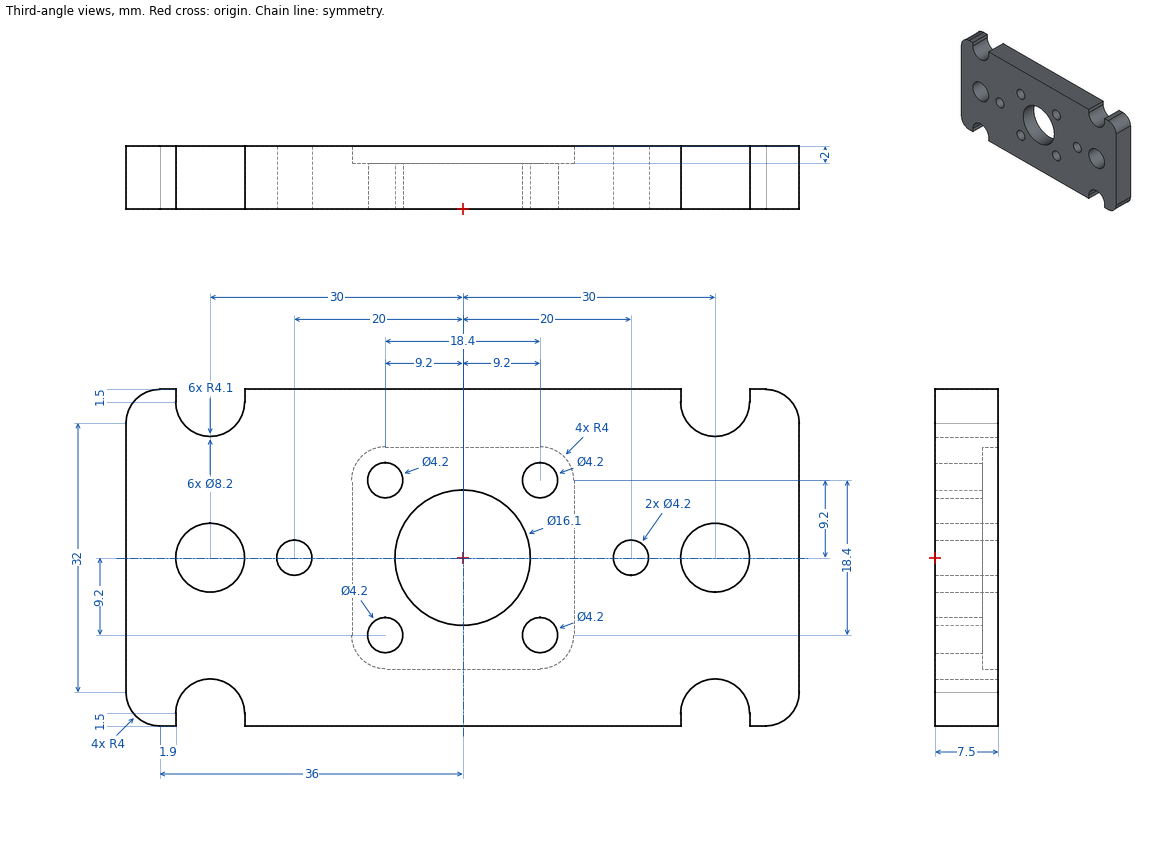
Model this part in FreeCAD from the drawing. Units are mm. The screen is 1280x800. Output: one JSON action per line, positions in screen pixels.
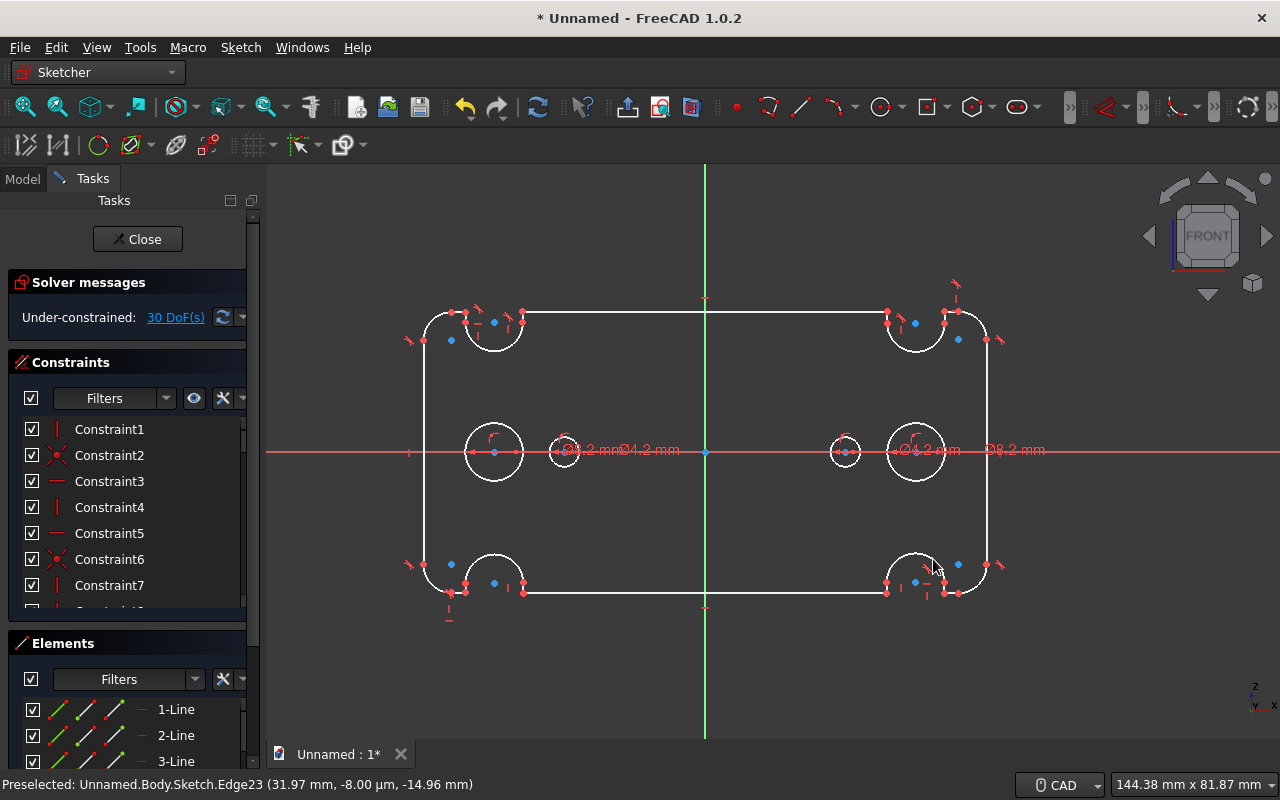
{"action": "scroll", "coordinate": [887, 588], "scroll_direction": "up", "scroll_amount": 5}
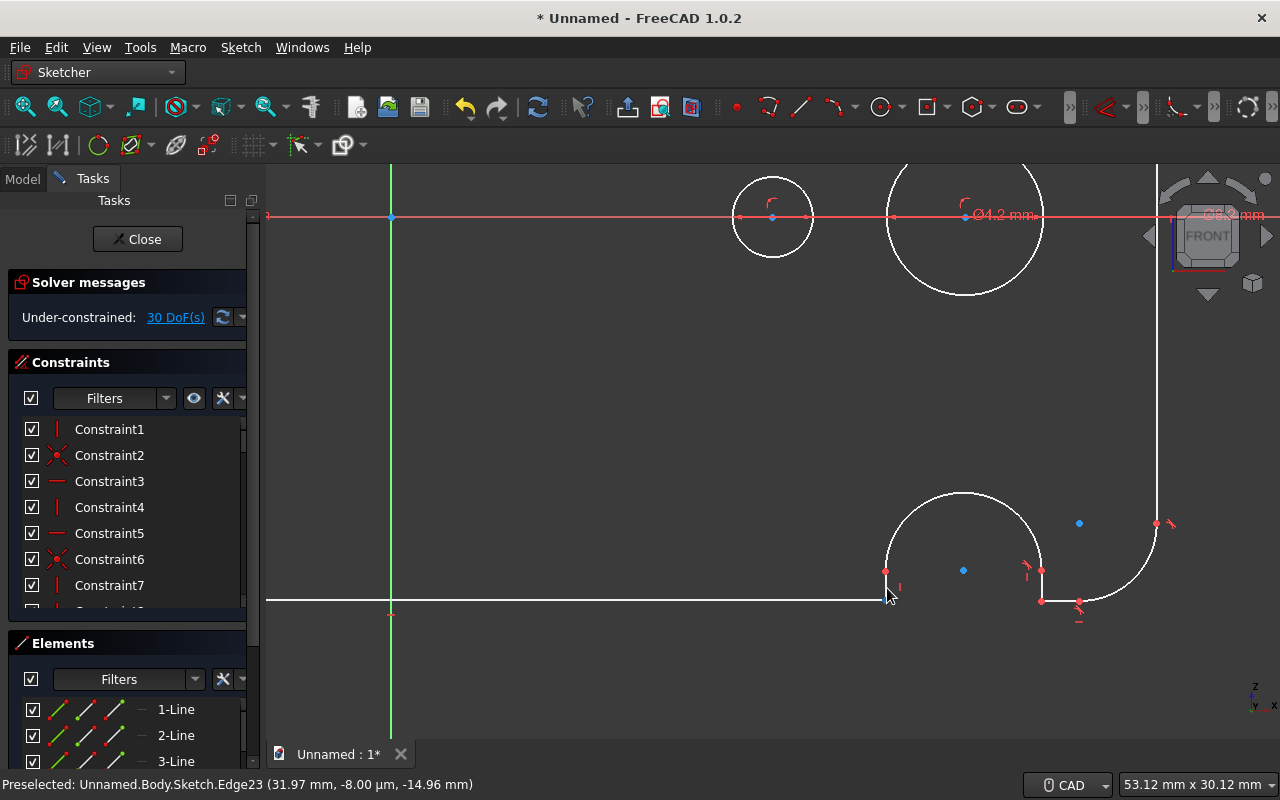
{"action": "left_click", "coordinate": [886, 586]}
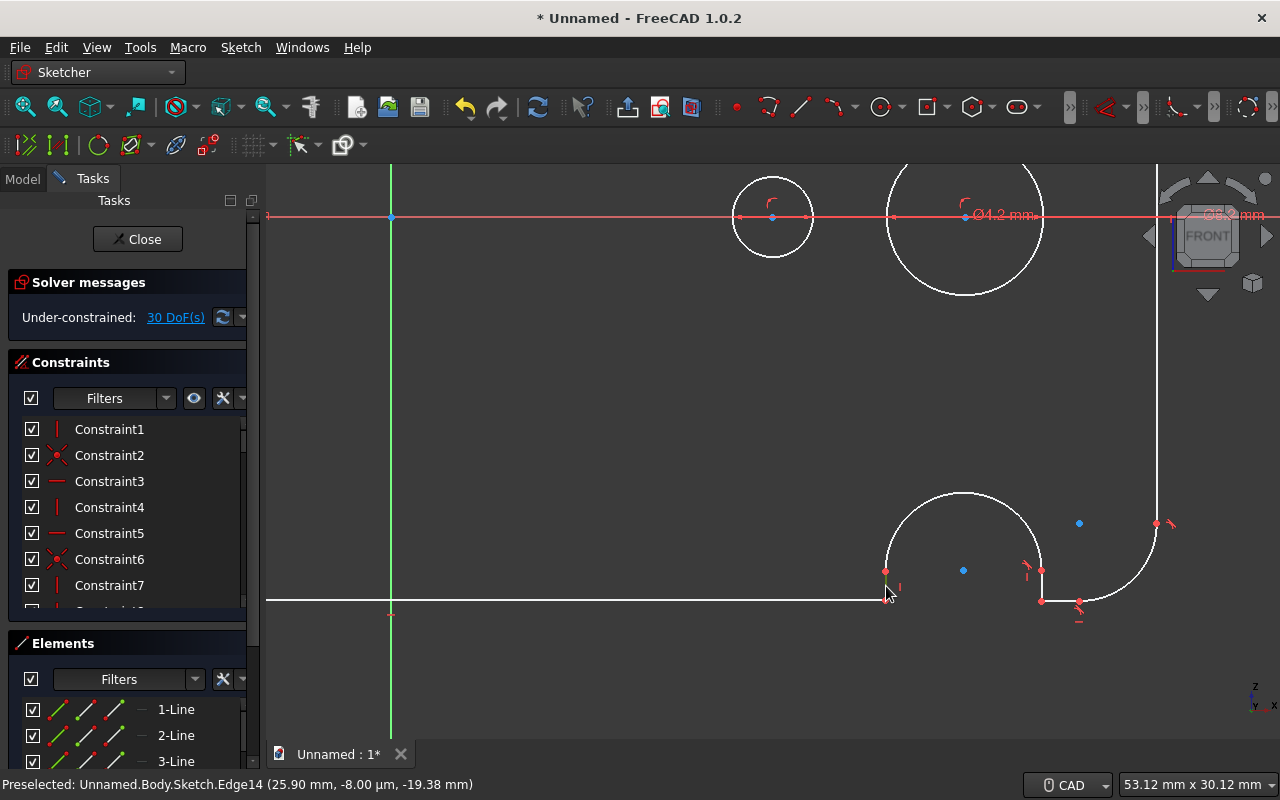
{"action": "left_click", "coordinate": [1009, 507]}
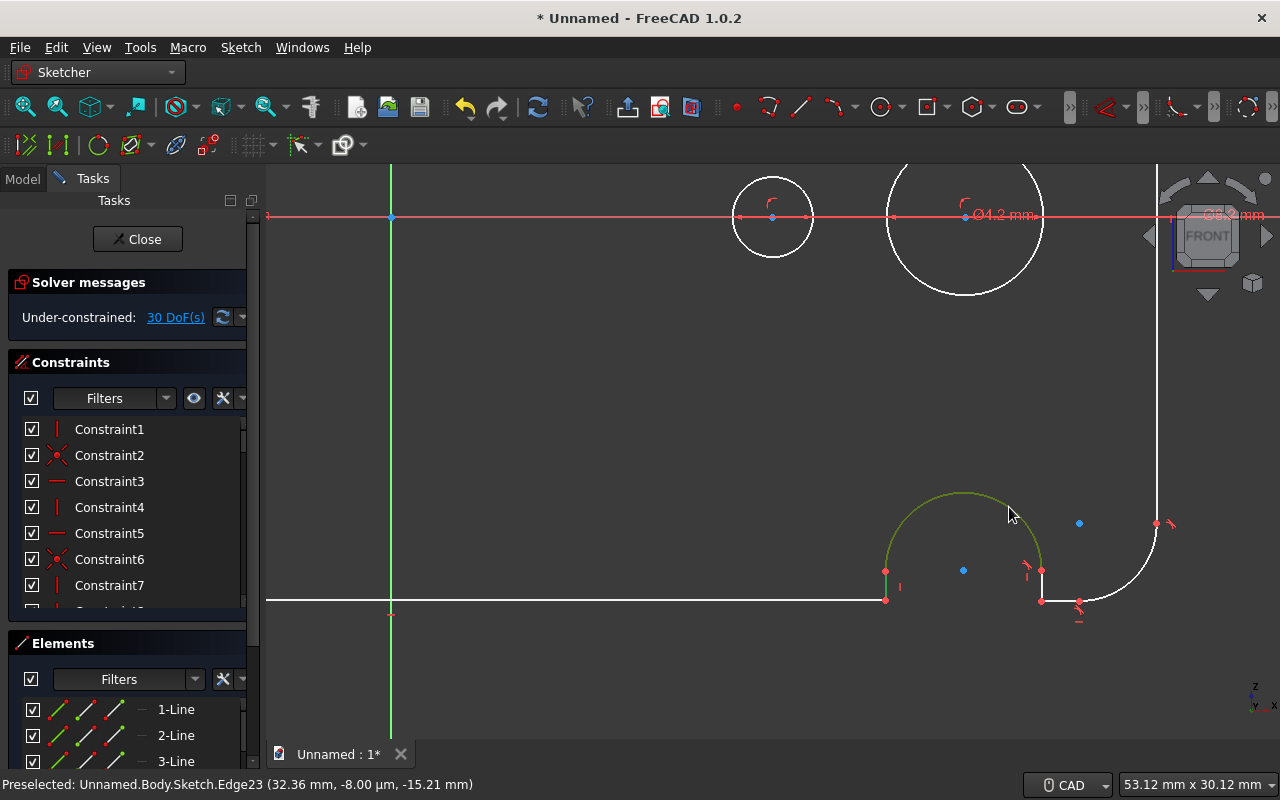
{"action": "key", "text": "t"}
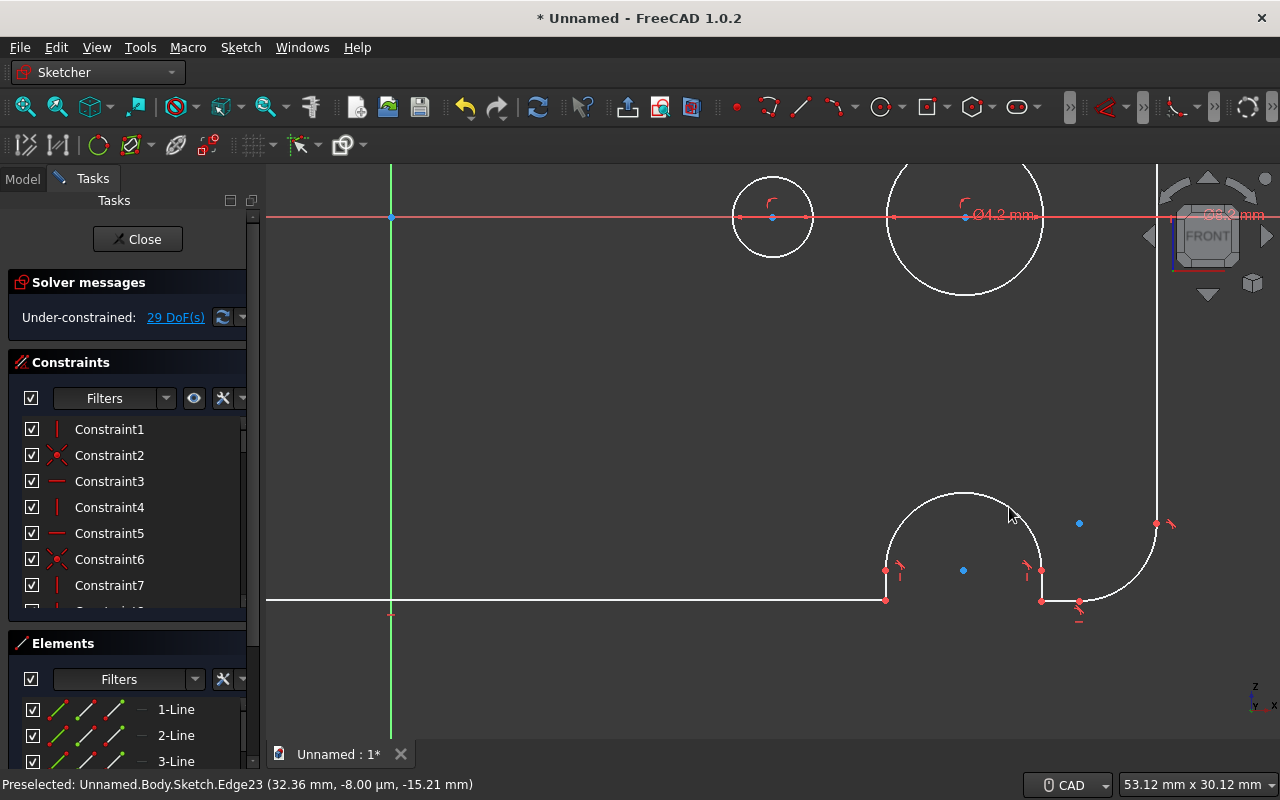
{"action": "scroll", "coordinate": [887, 588], "scroll_direction": "down", "scroll_amount": 5}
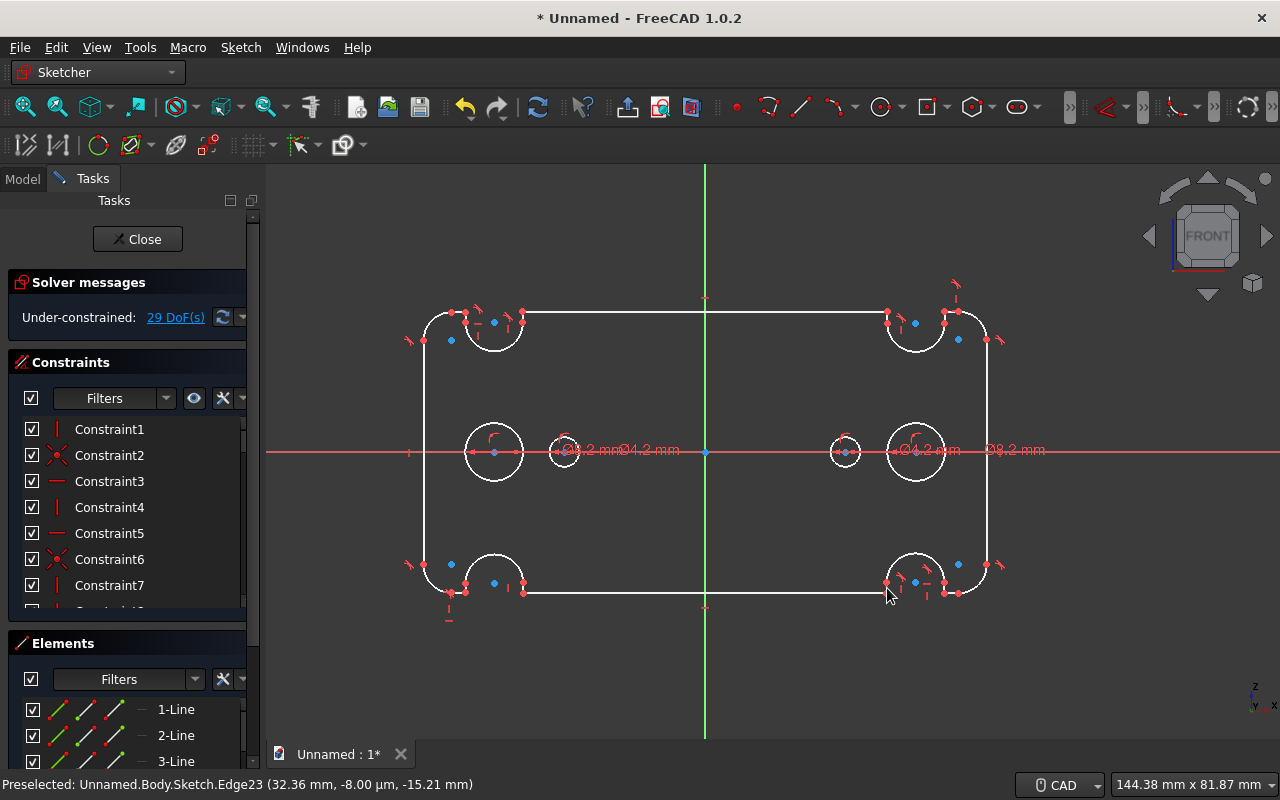
{"action": "scroll", "coordinate": [523, 589], "scroll_direction": "up", "scroll_amount": 6}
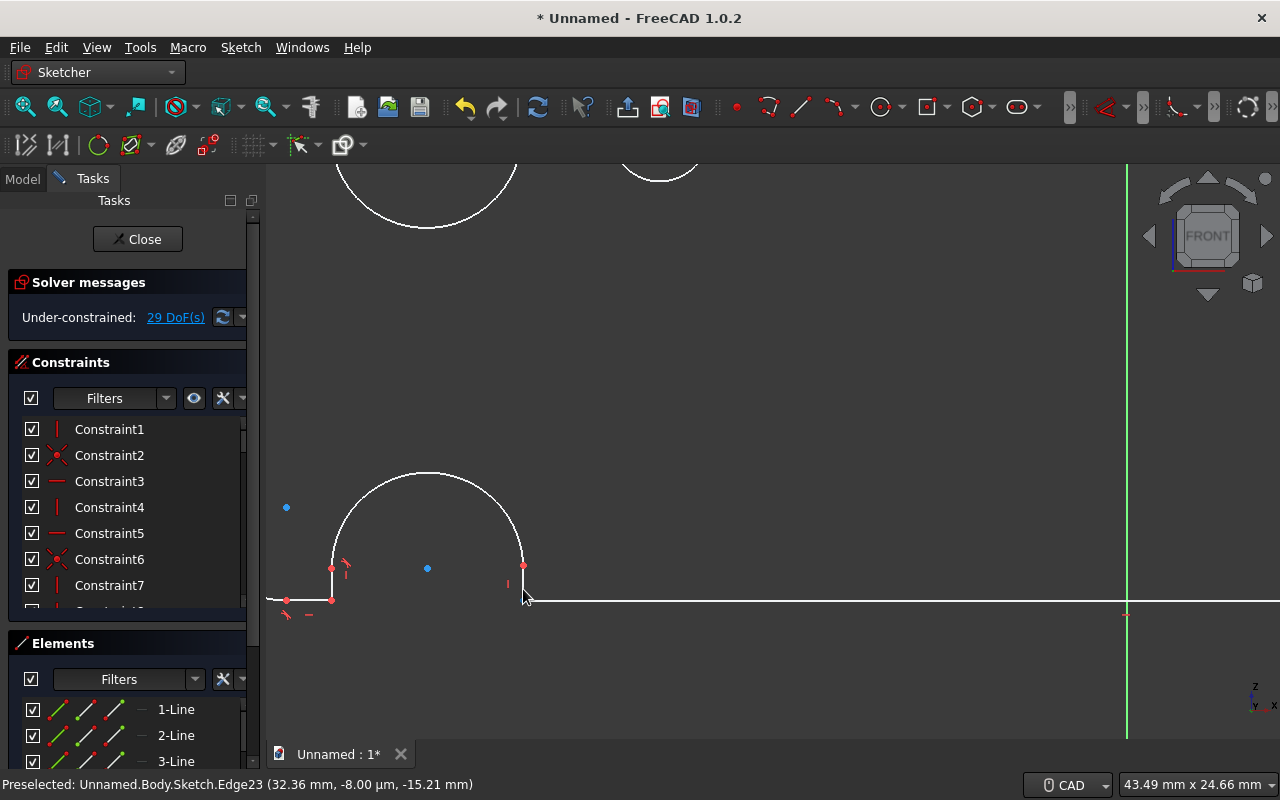
{"action": "left_click", "coordinate": [523, 587]}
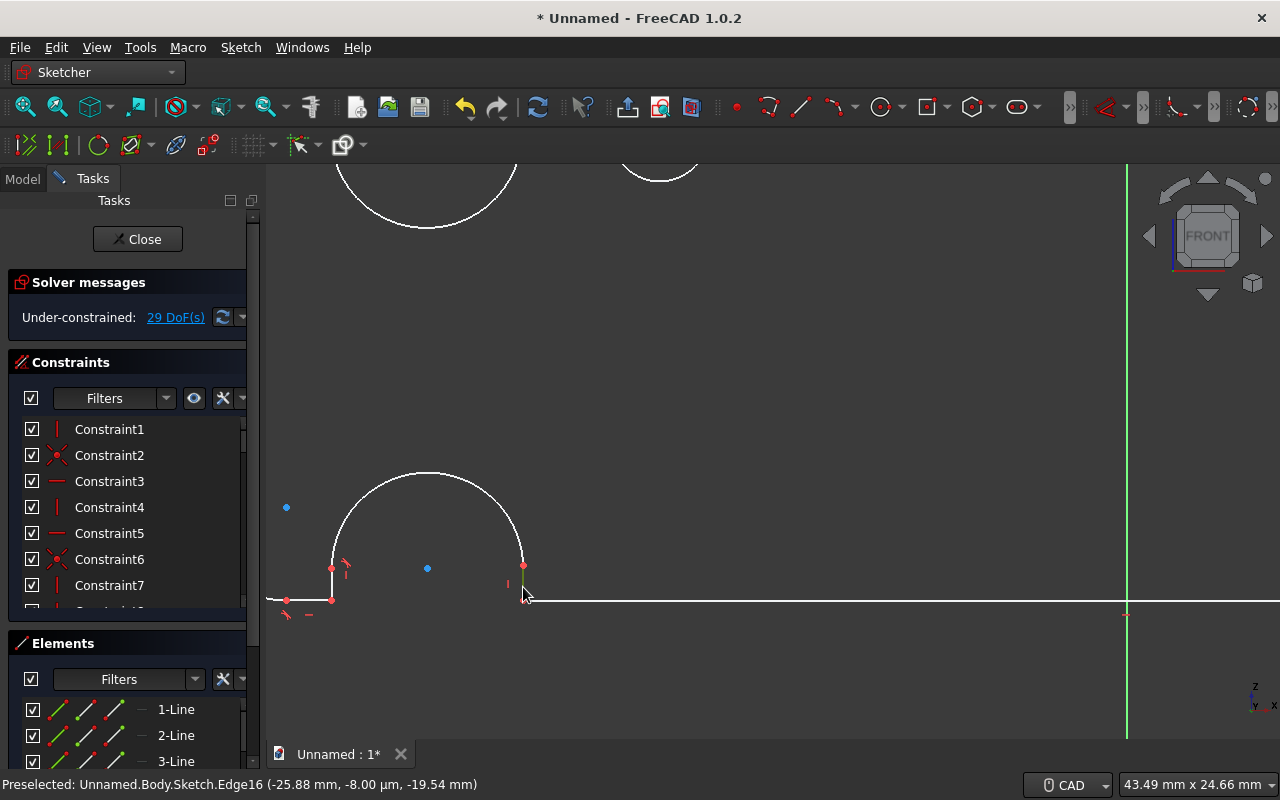
{"action": "scroll", "coordinate": [523, 589], "scroll_direction": "down", "scroll_amount": 6}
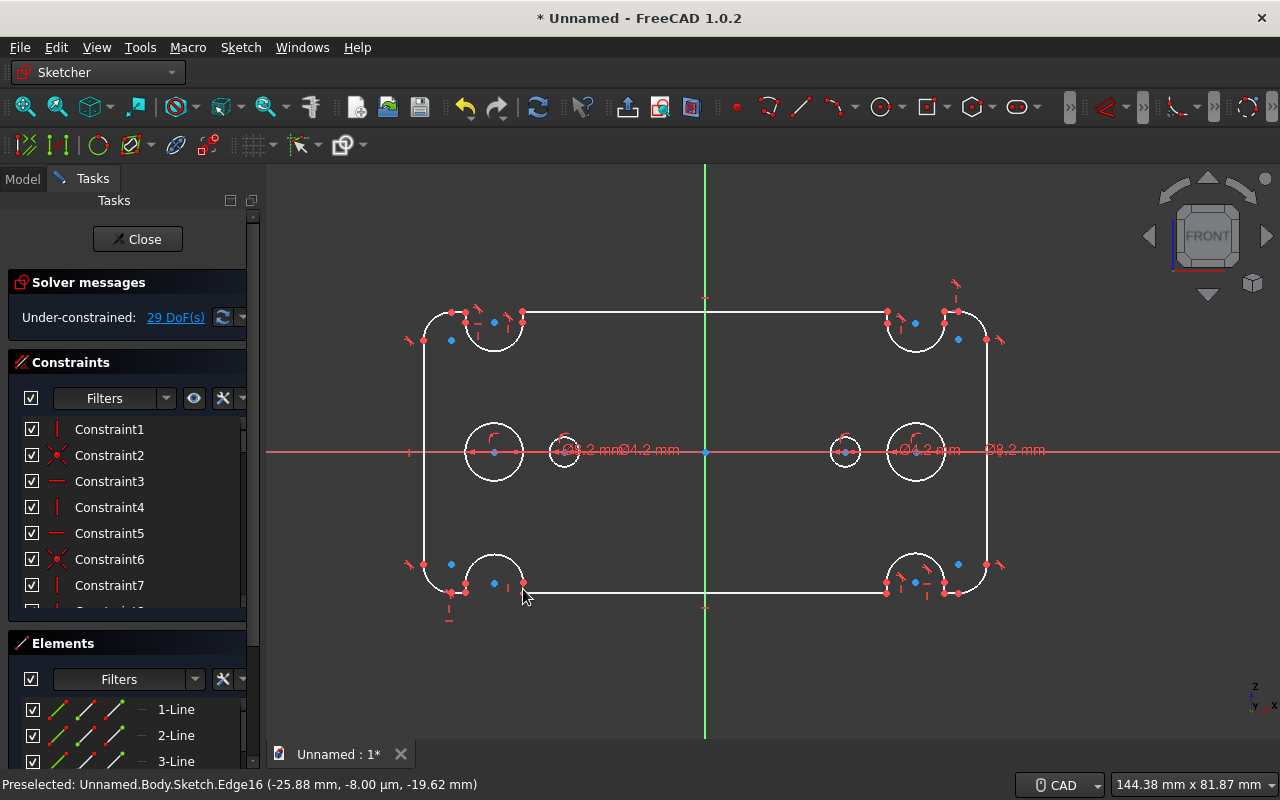
{"action": "left_click", "coordinate": [511, 560]}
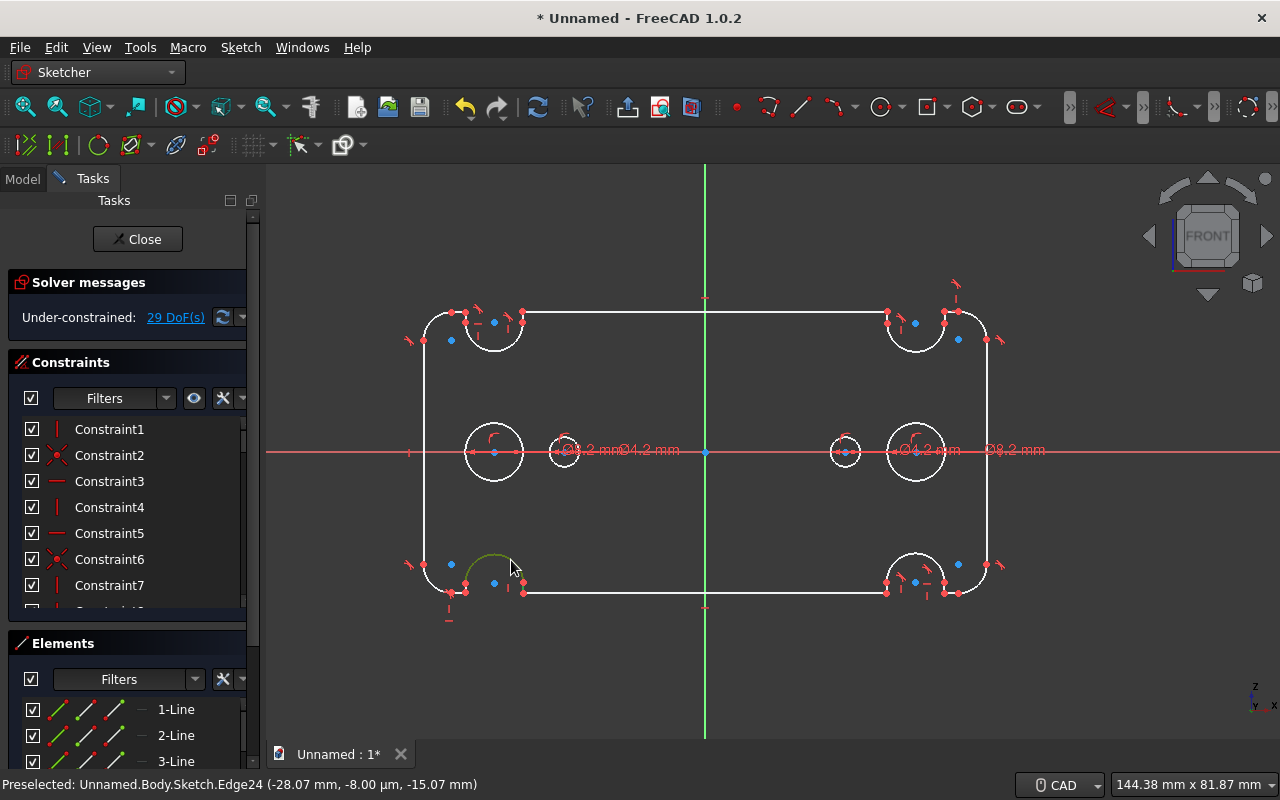
{"action": "key", "text": "t"}